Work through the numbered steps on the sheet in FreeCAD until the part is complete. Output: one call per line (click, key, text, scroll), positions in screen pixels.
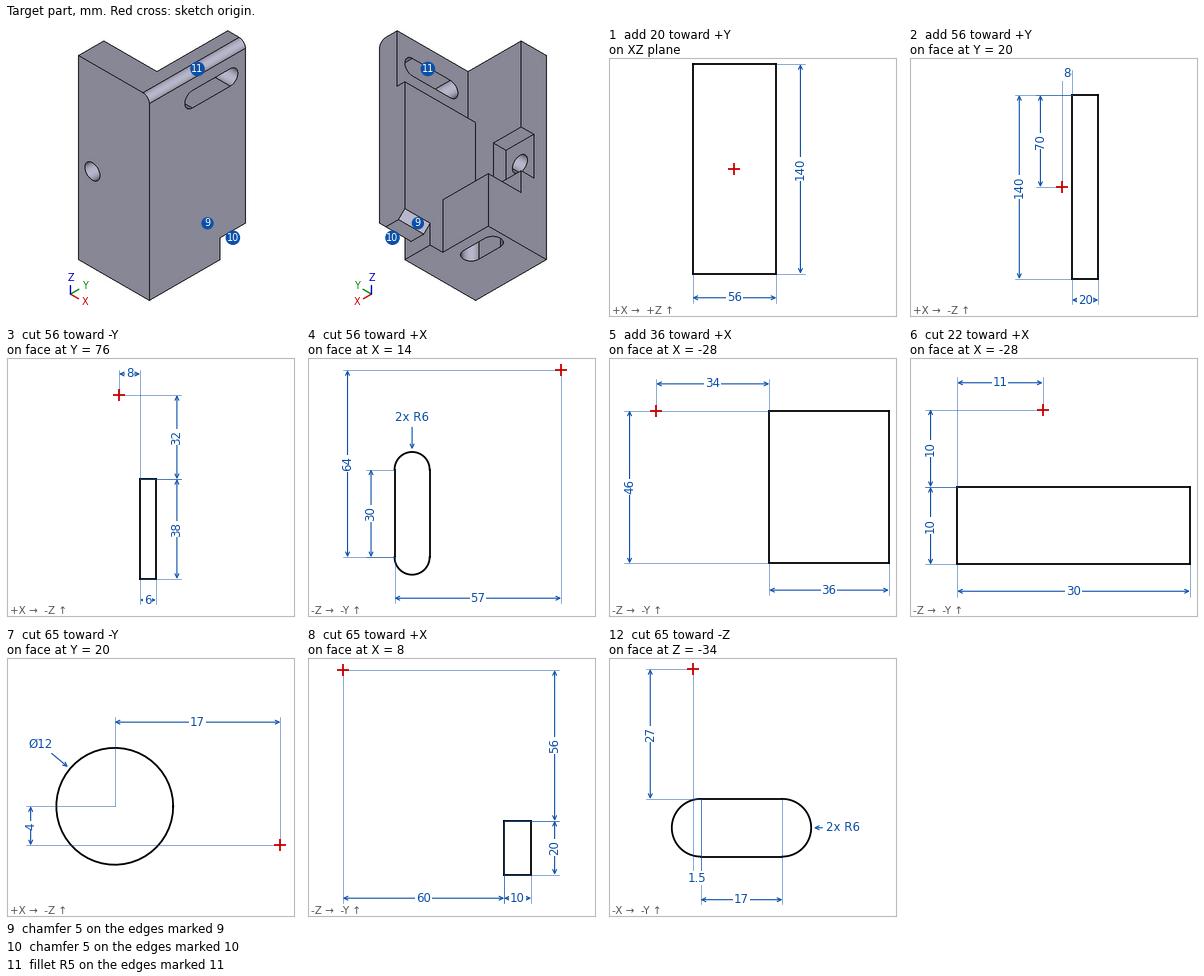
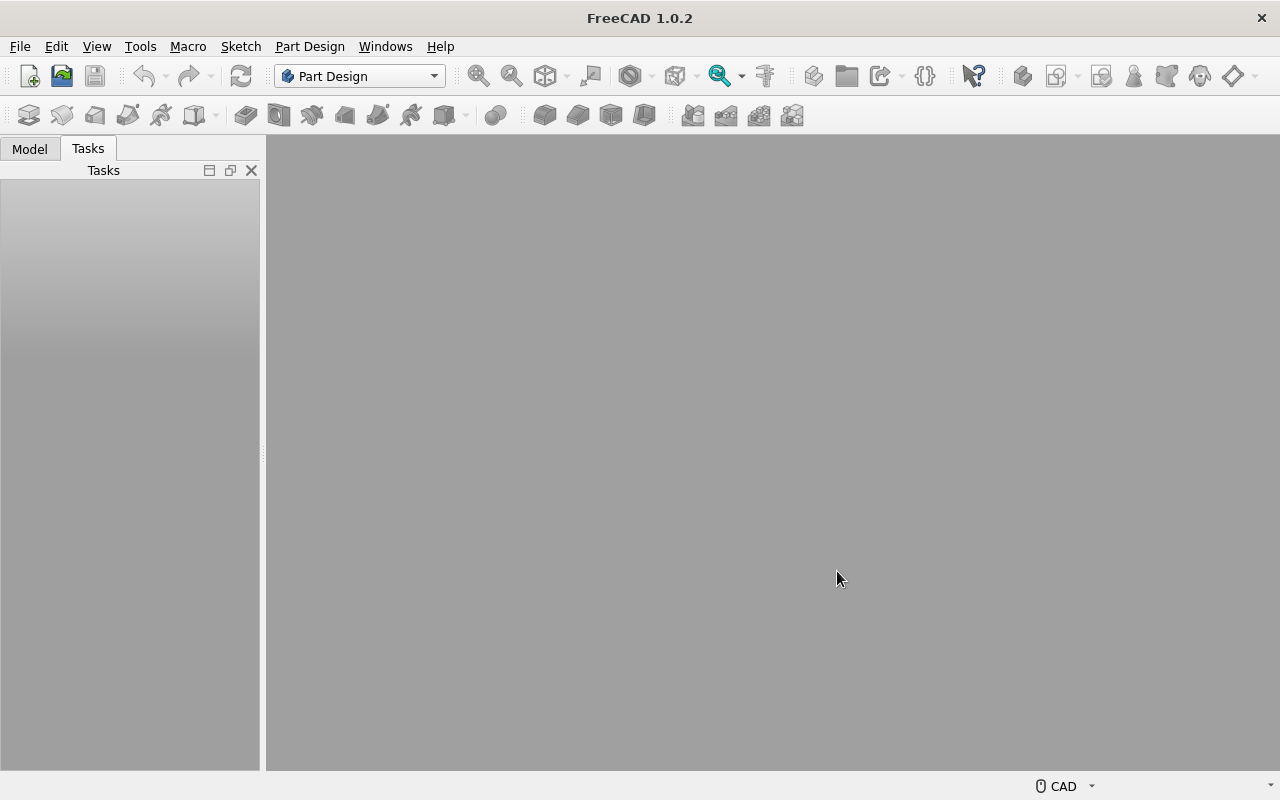
click(29, 76)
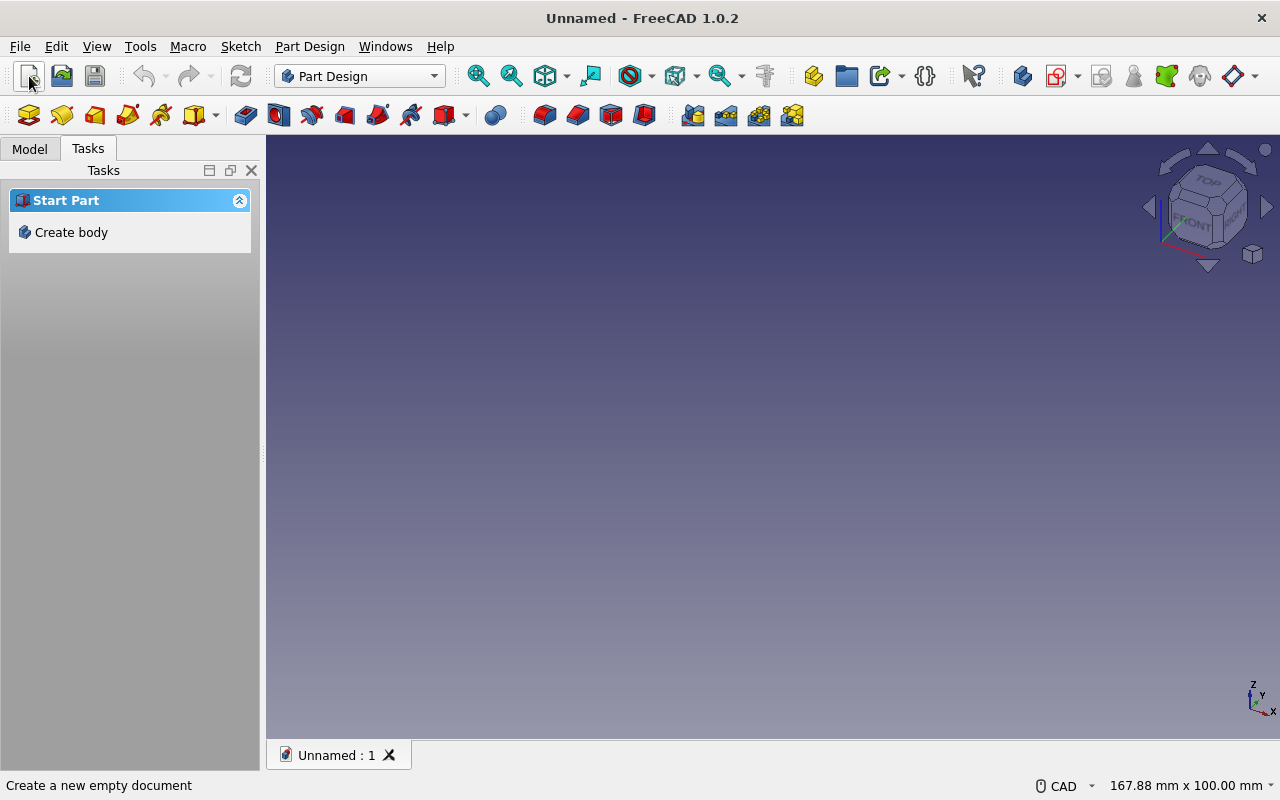
click(1056, 76)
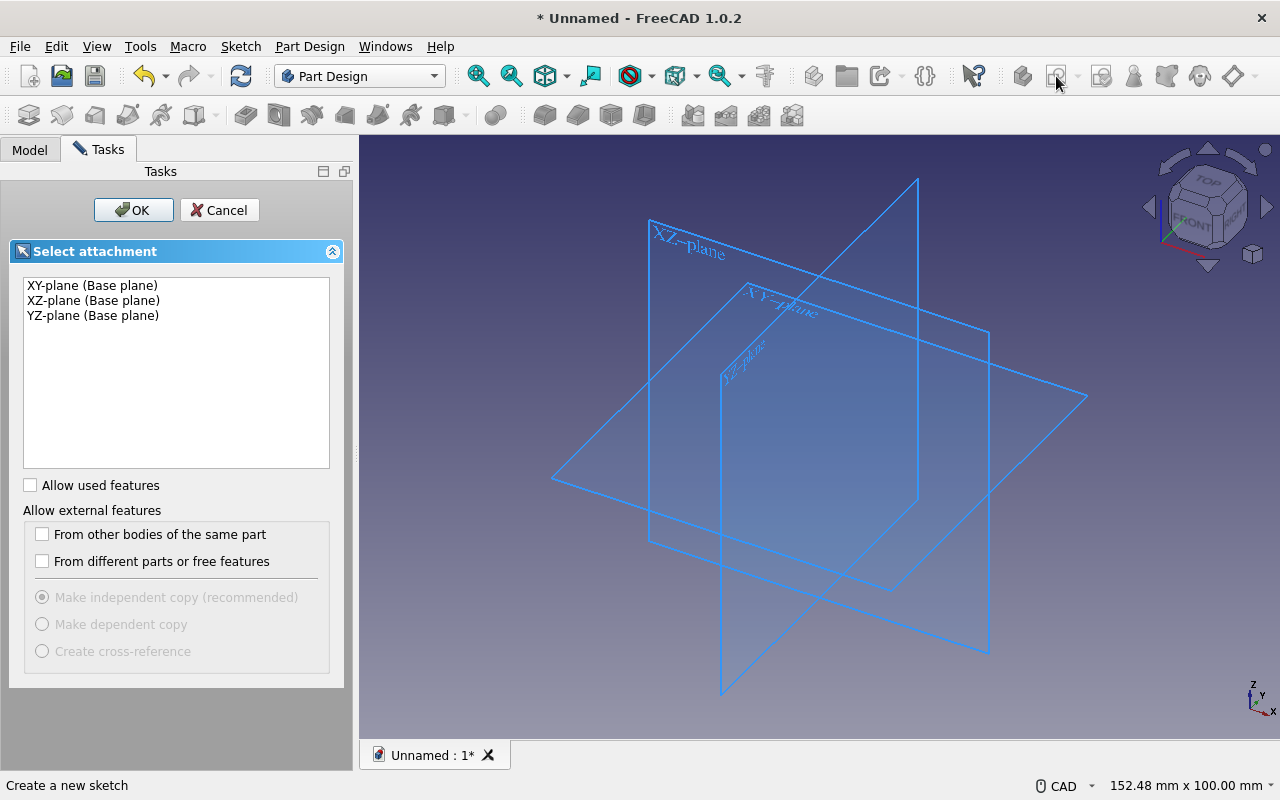
click(84, 300)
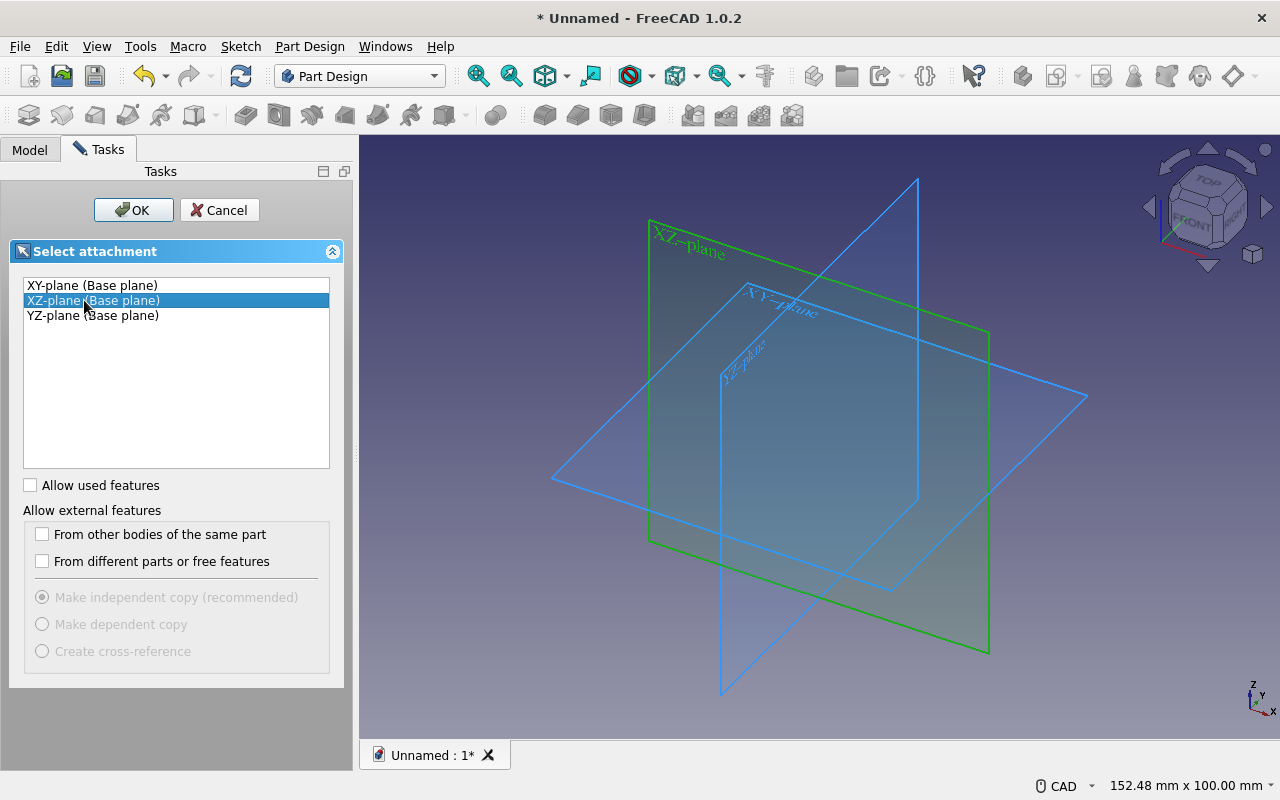
click(134, 210)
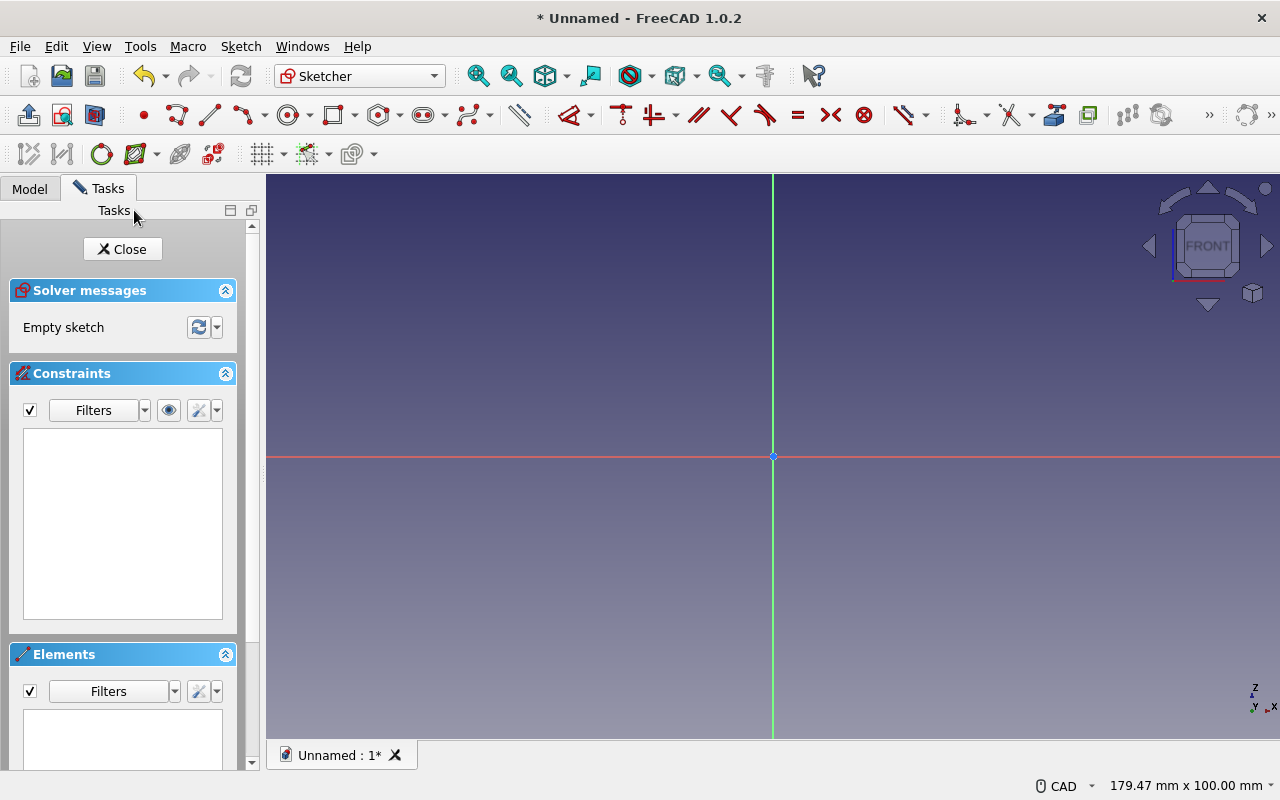
scroll(649, 456, down, 4)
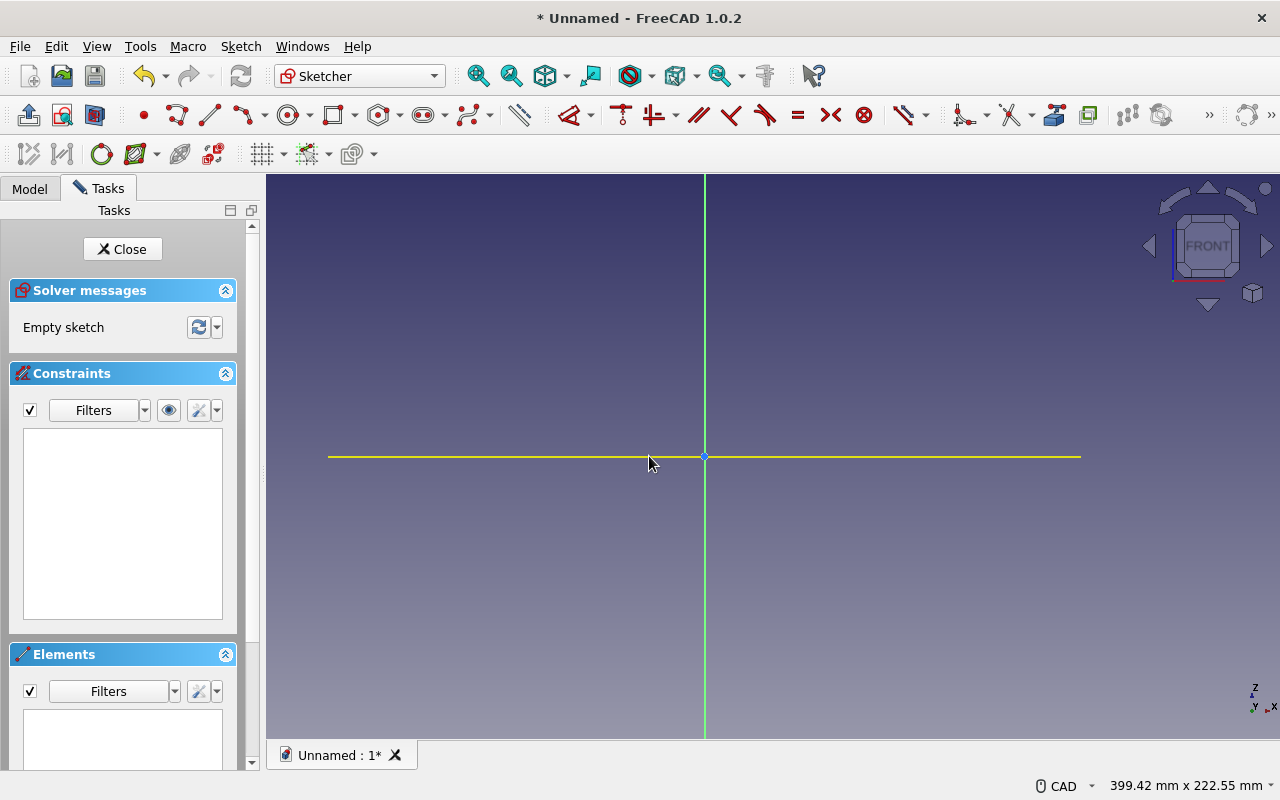
key(g)
key(v)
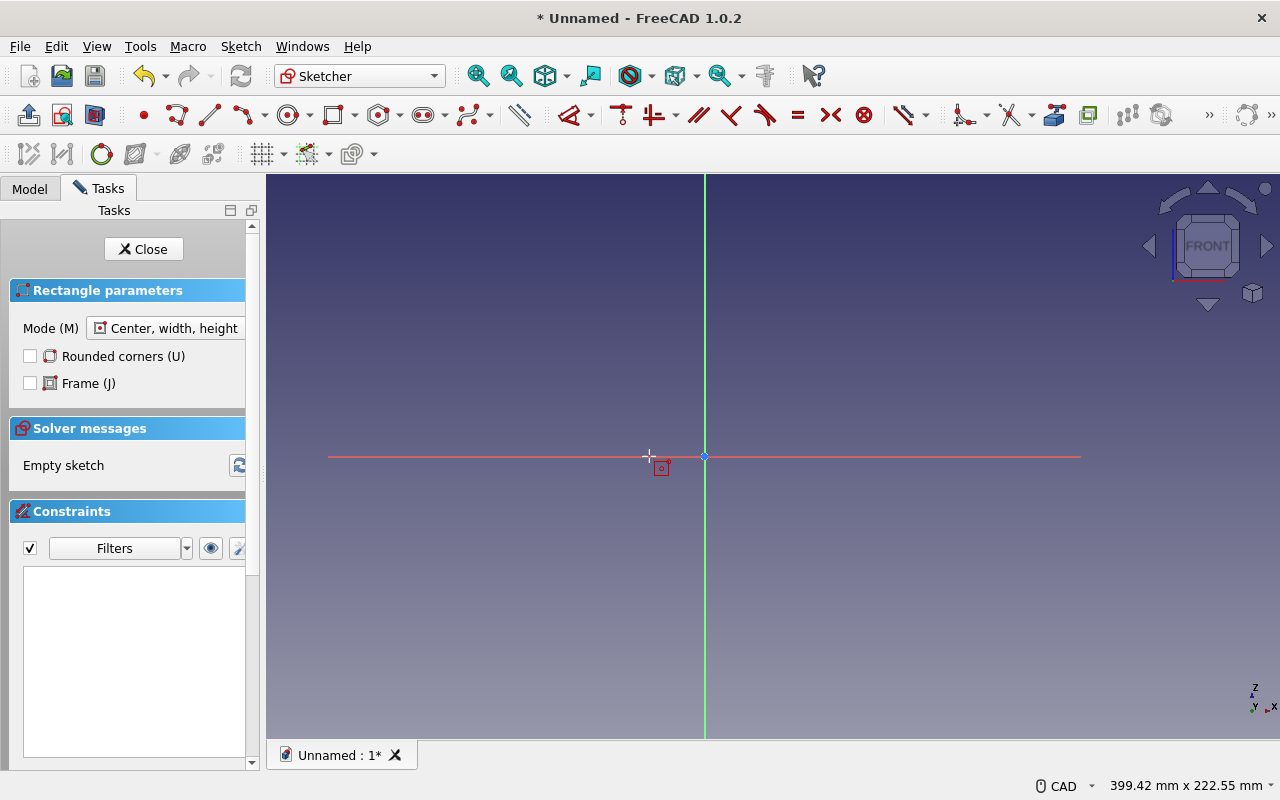
click(705, 456)
click(776, 279)
key(Escape)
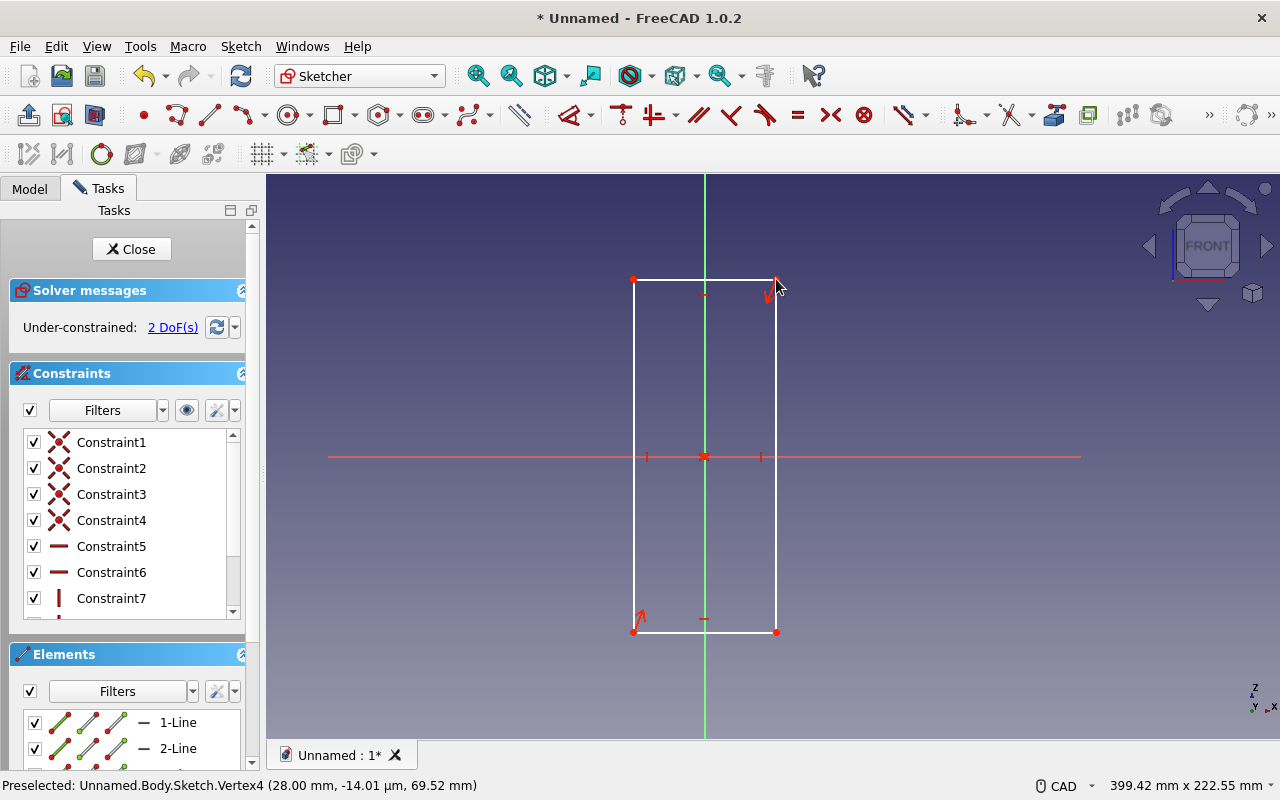
click(568, 116)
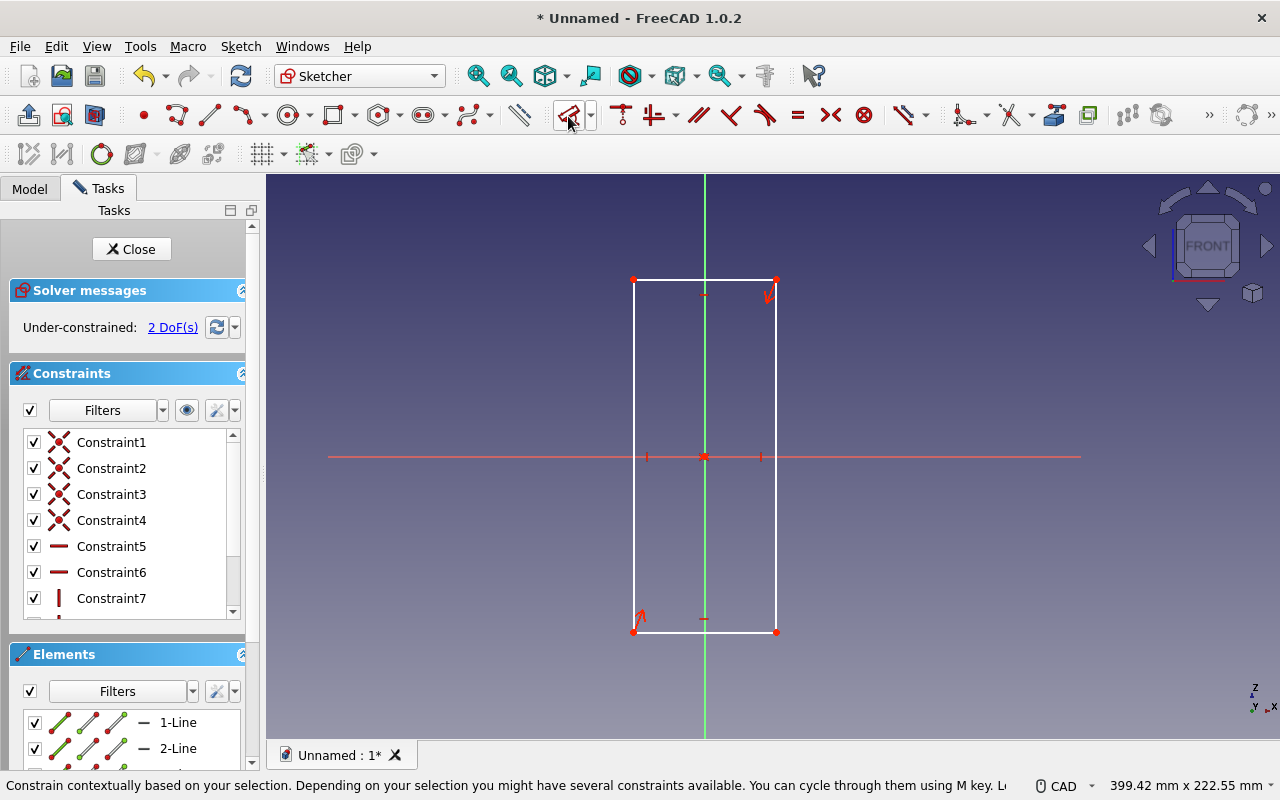
click(676, 633)
click(672, 667)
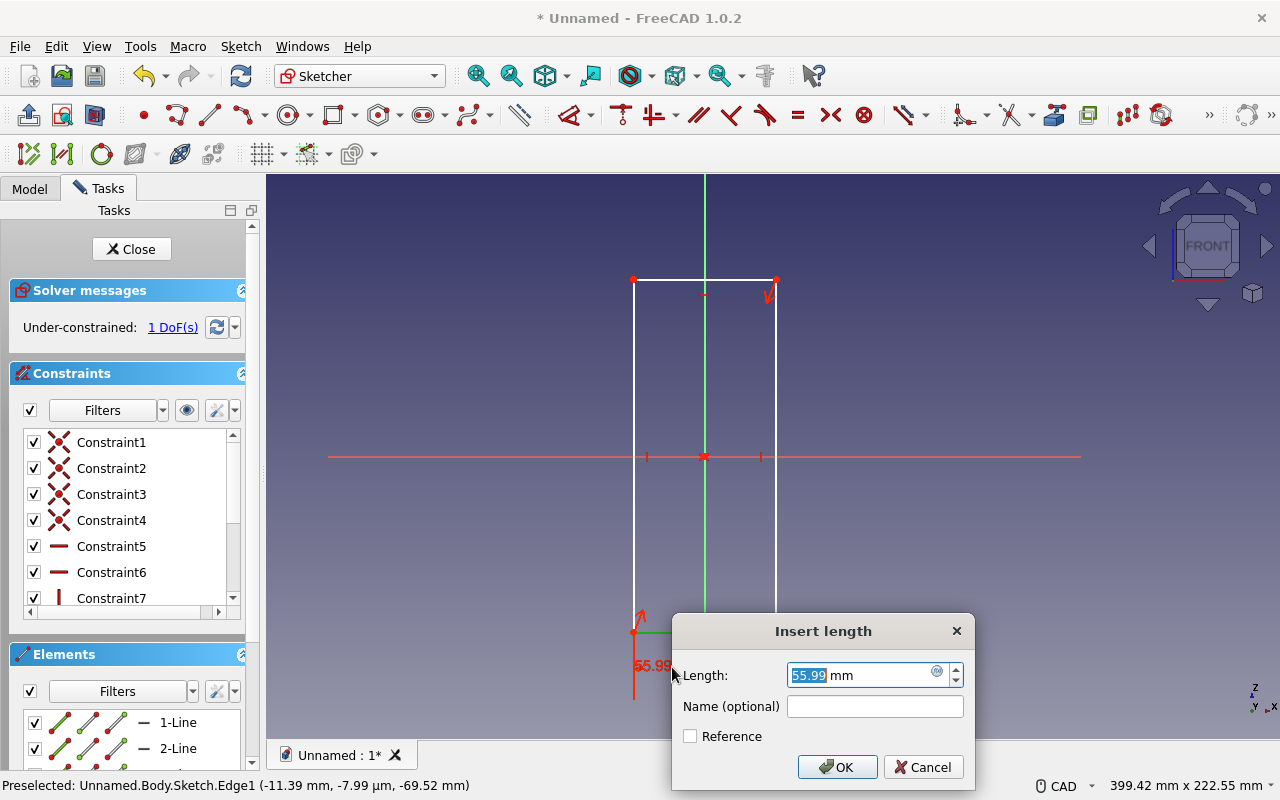
text(56)
key(Return)